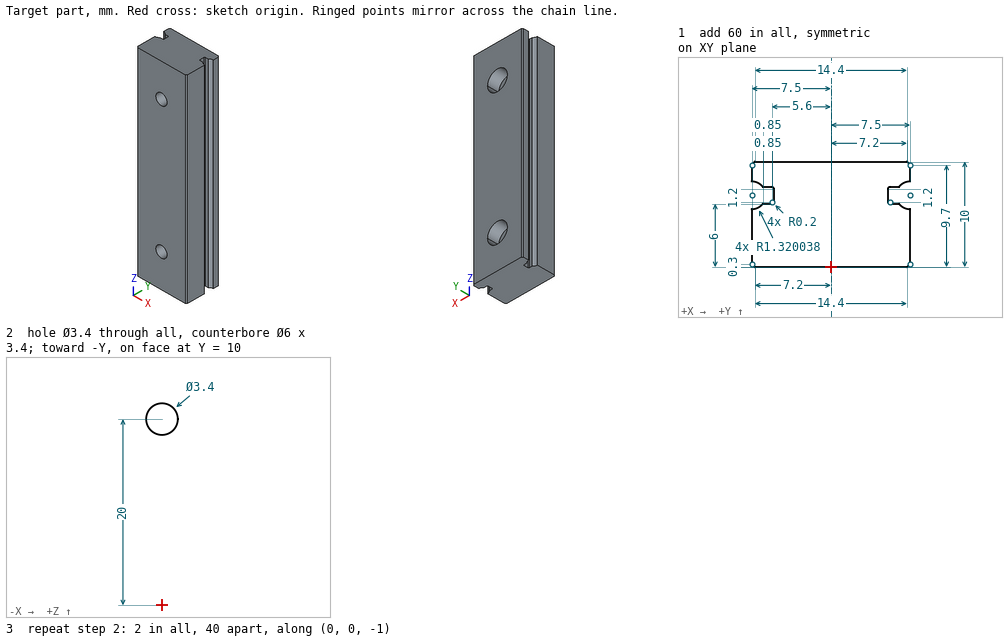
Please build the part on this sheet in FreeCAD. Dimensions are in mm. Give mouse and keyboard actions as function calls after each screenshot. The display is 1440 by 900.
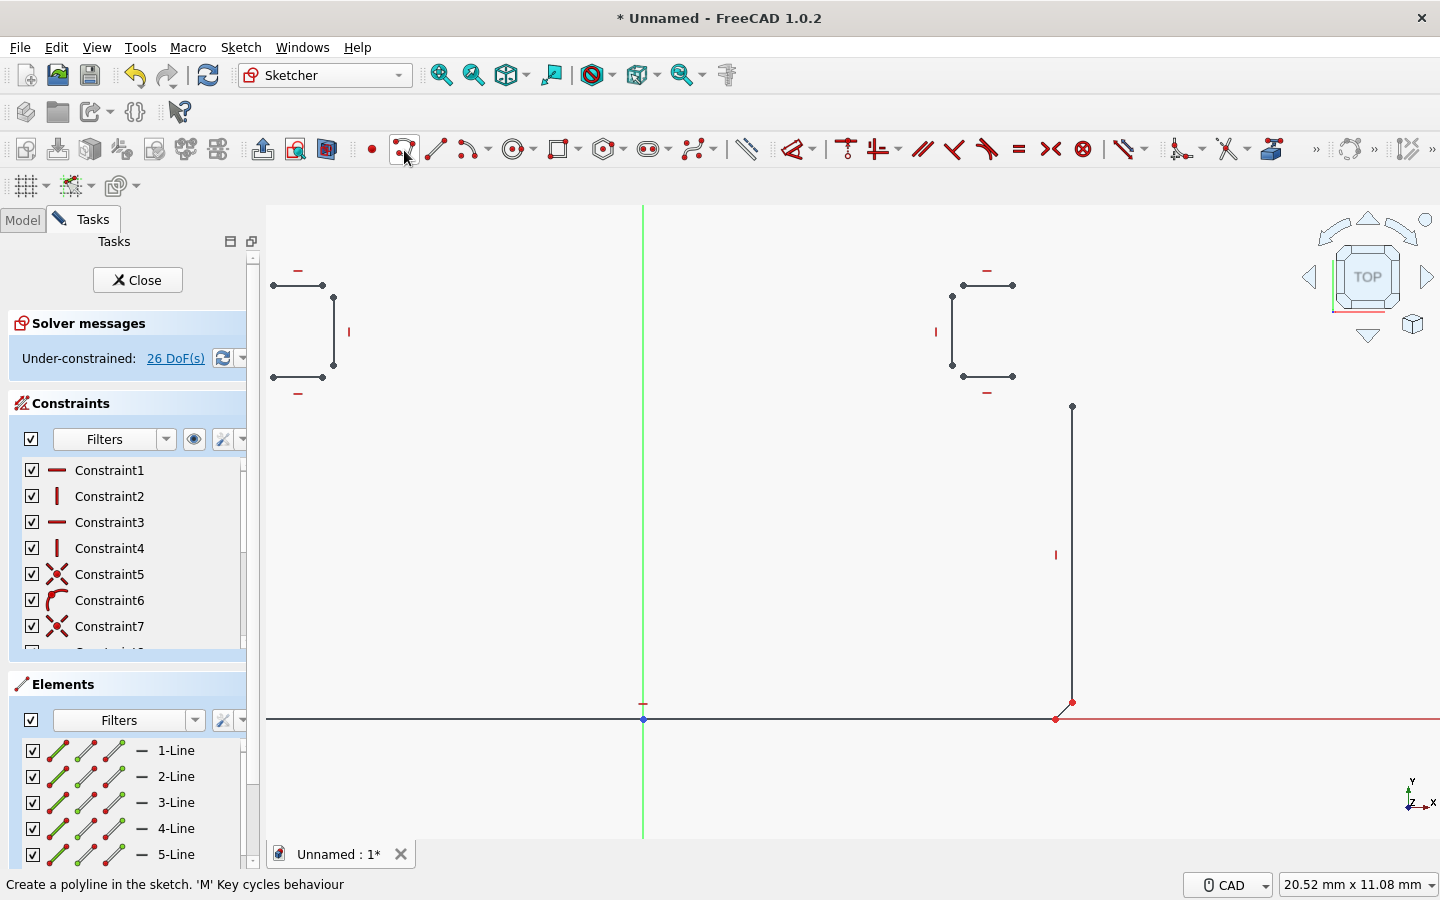
click(1072, 255)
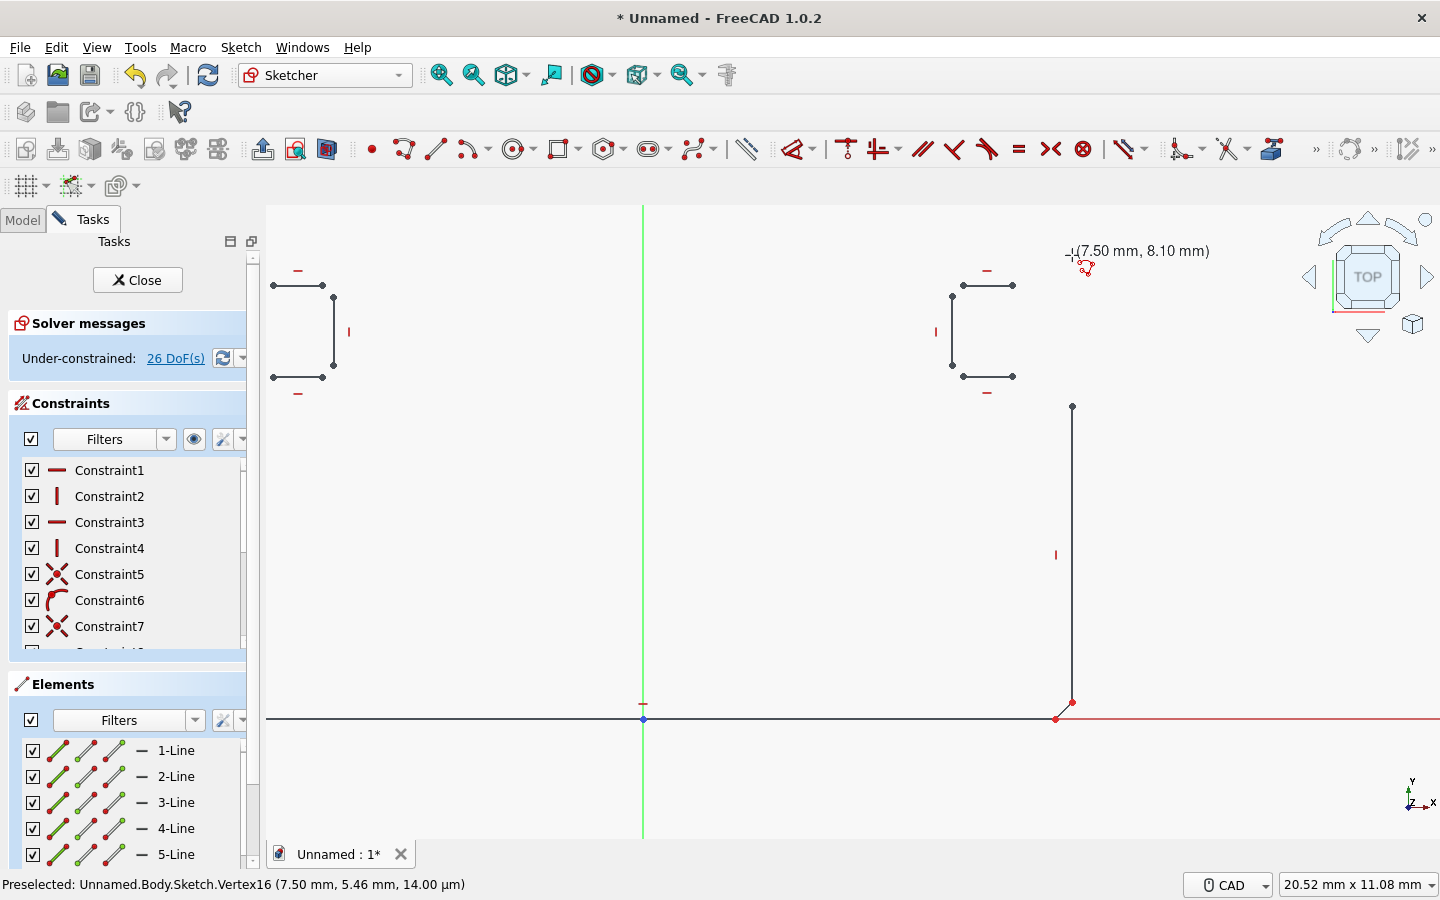
scroll(1072, 702, down, 2)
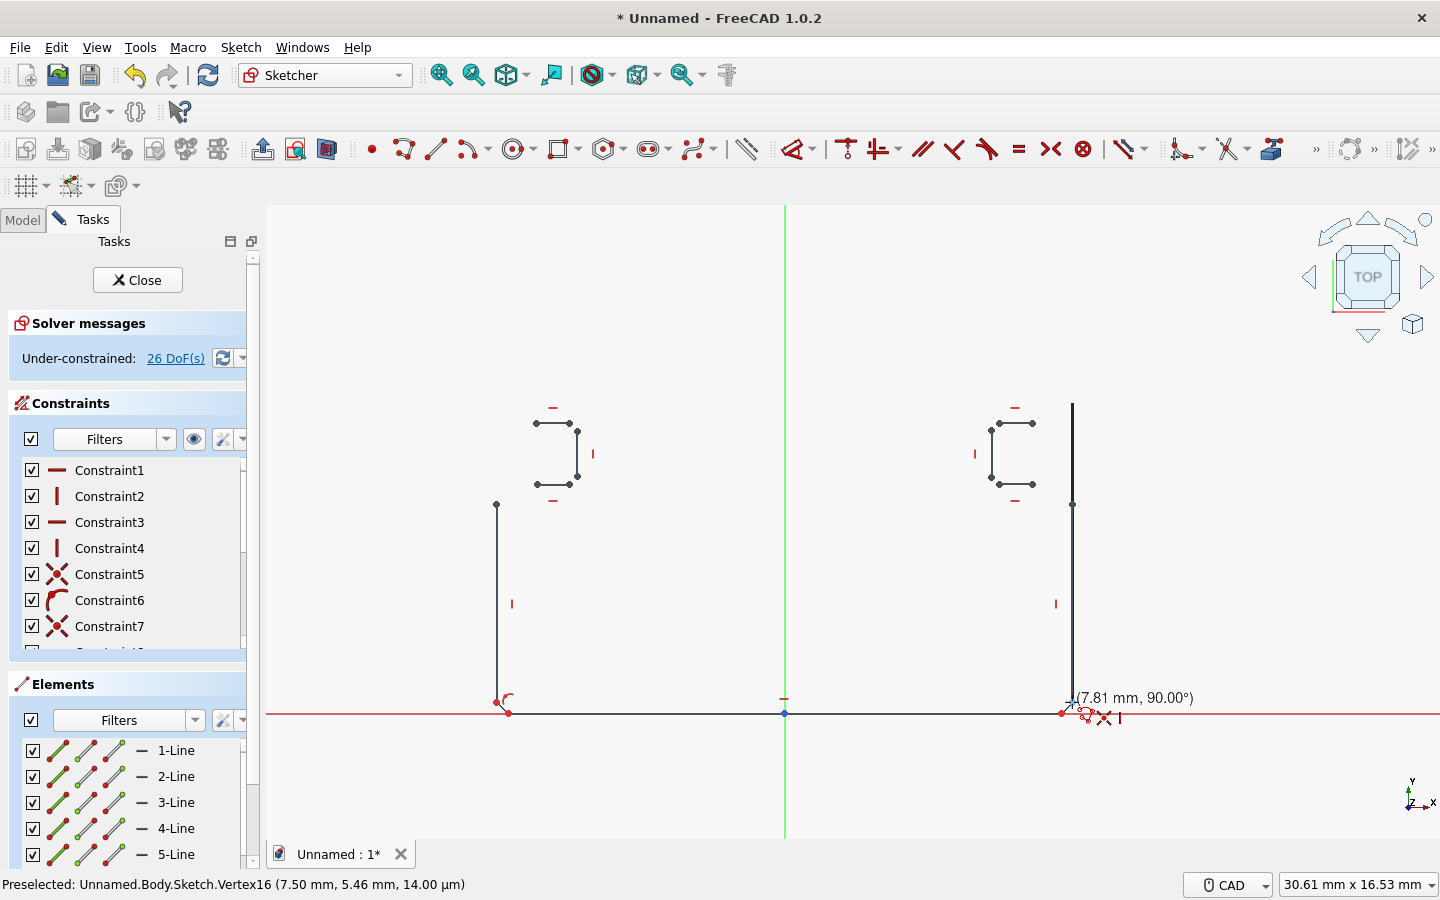
click(1072, 342)
click(1061, 330)
click(509, 330)
click(497, 342)
click(497, 403)
right_click(497, 403)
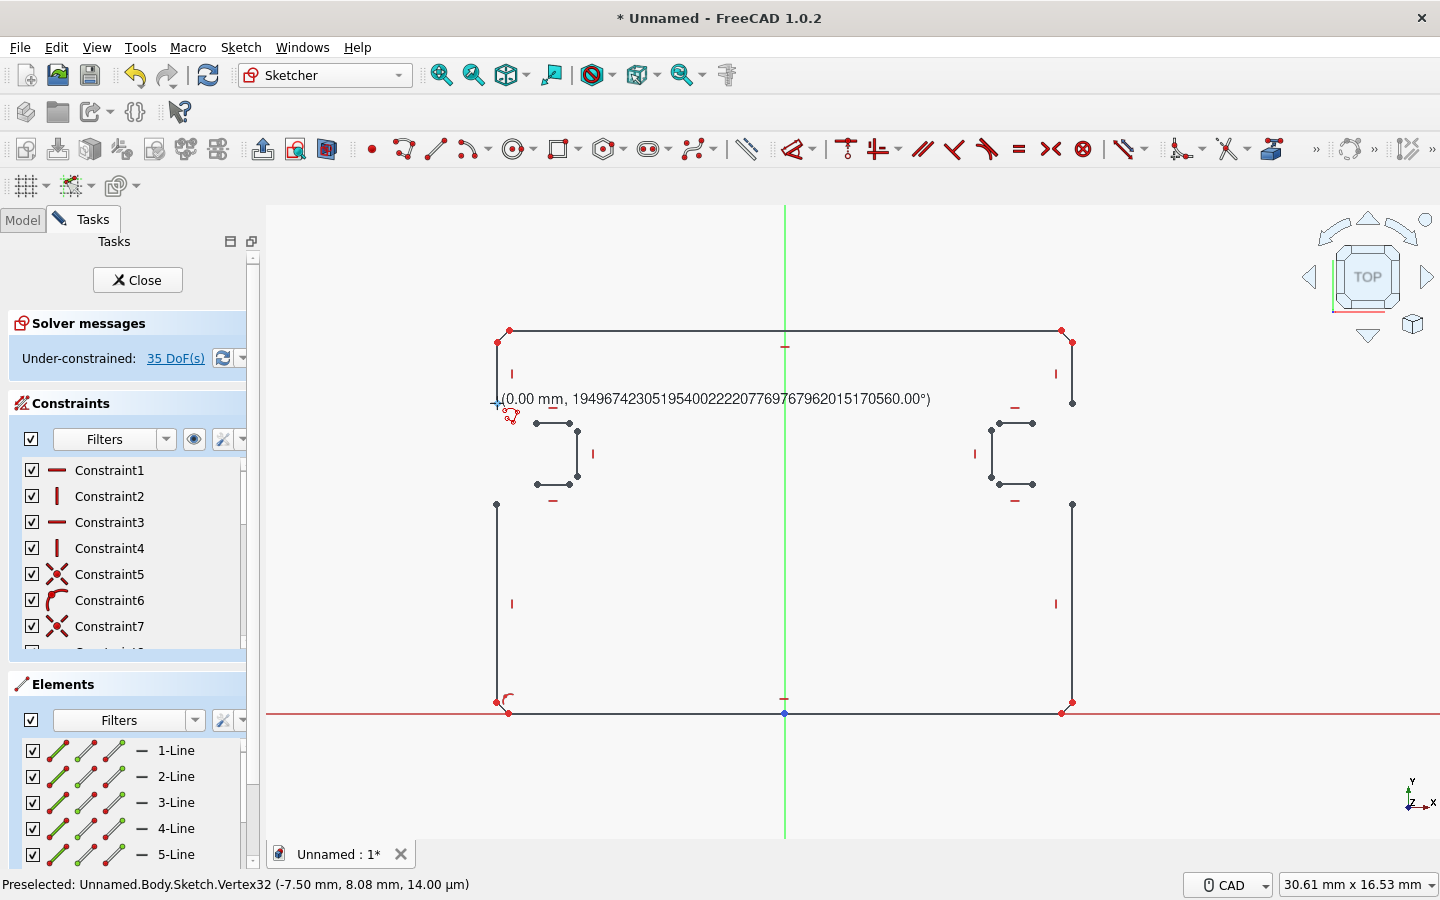
click(490, 150)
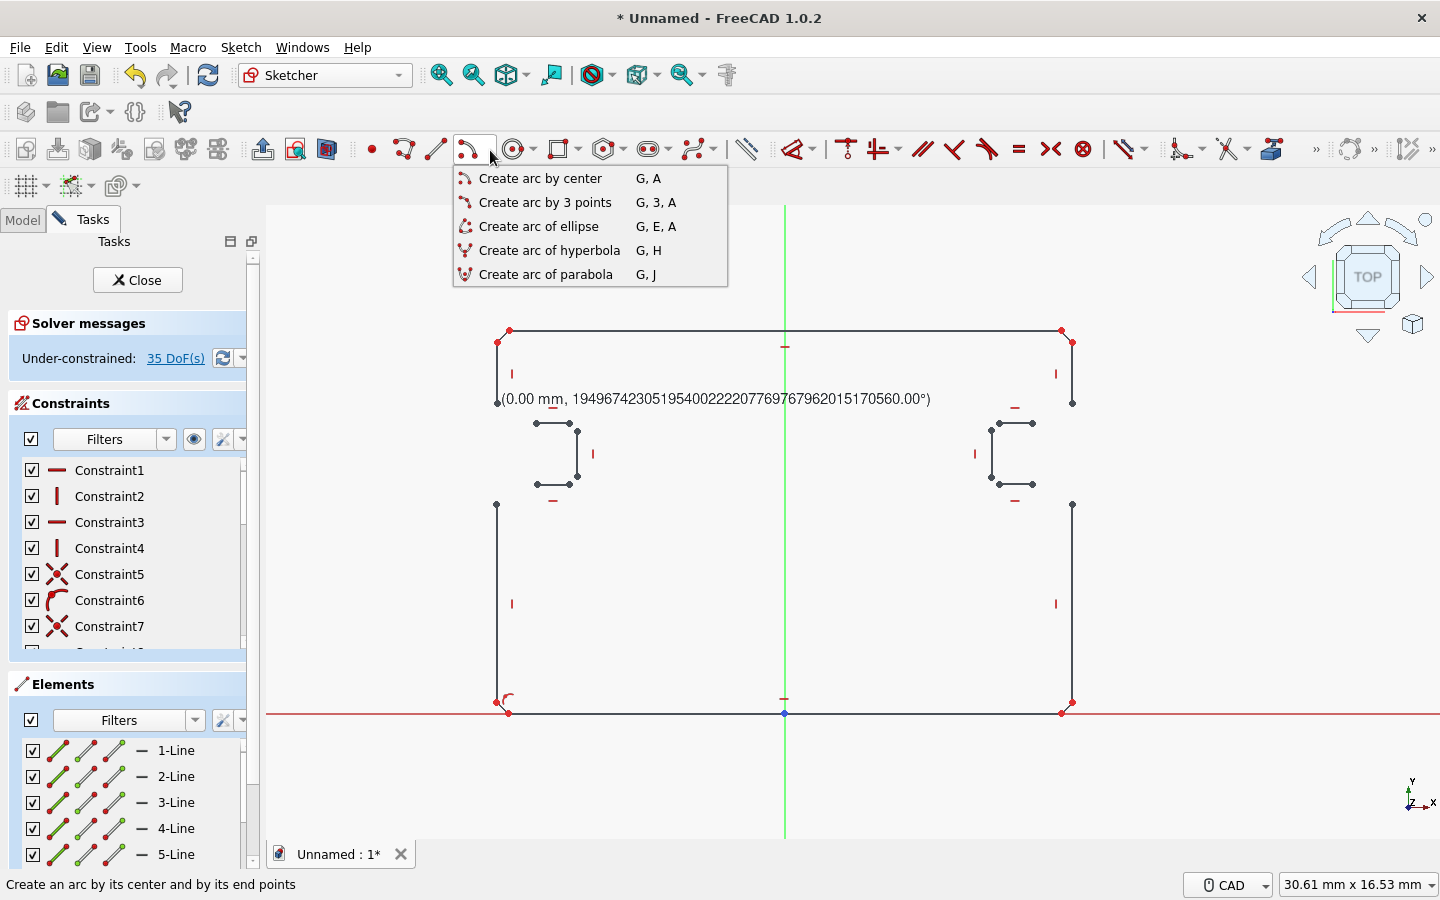
click(590, 202)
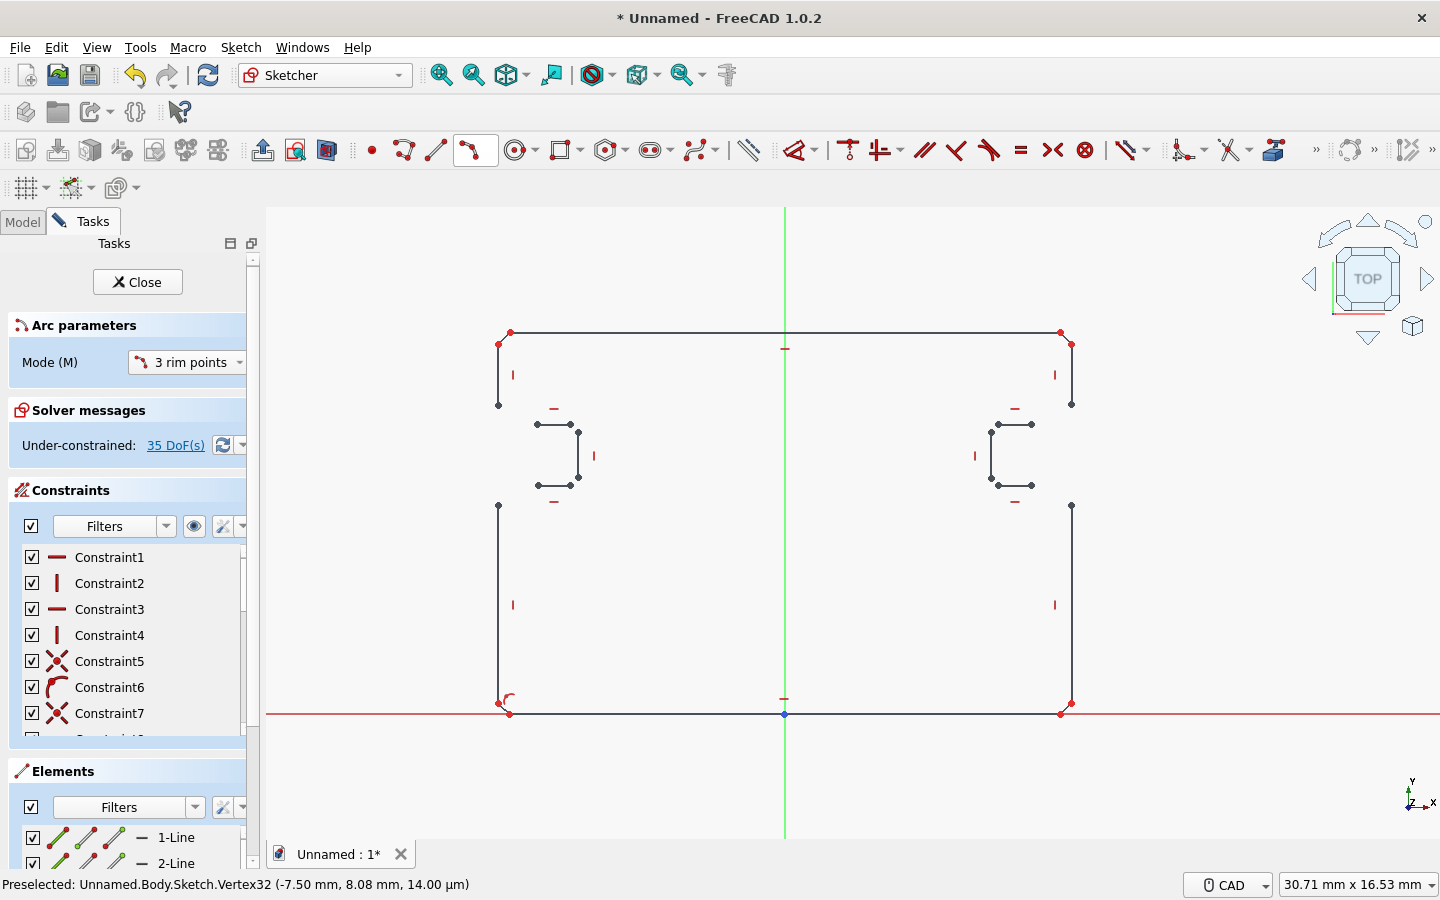
scroll(571, 424, up, 2)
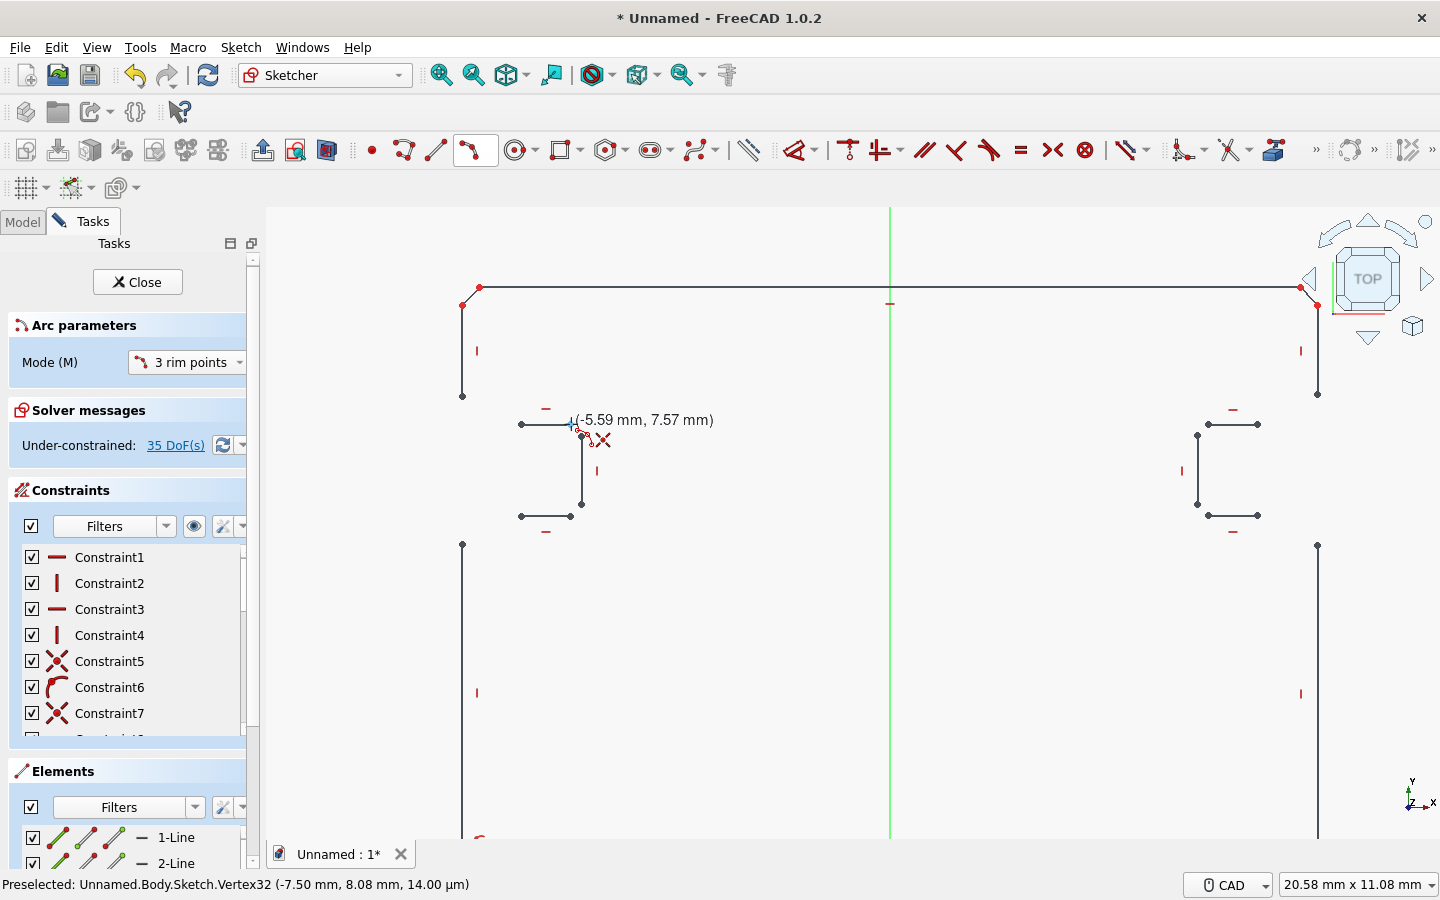
click(571, 425)
click(582, 436)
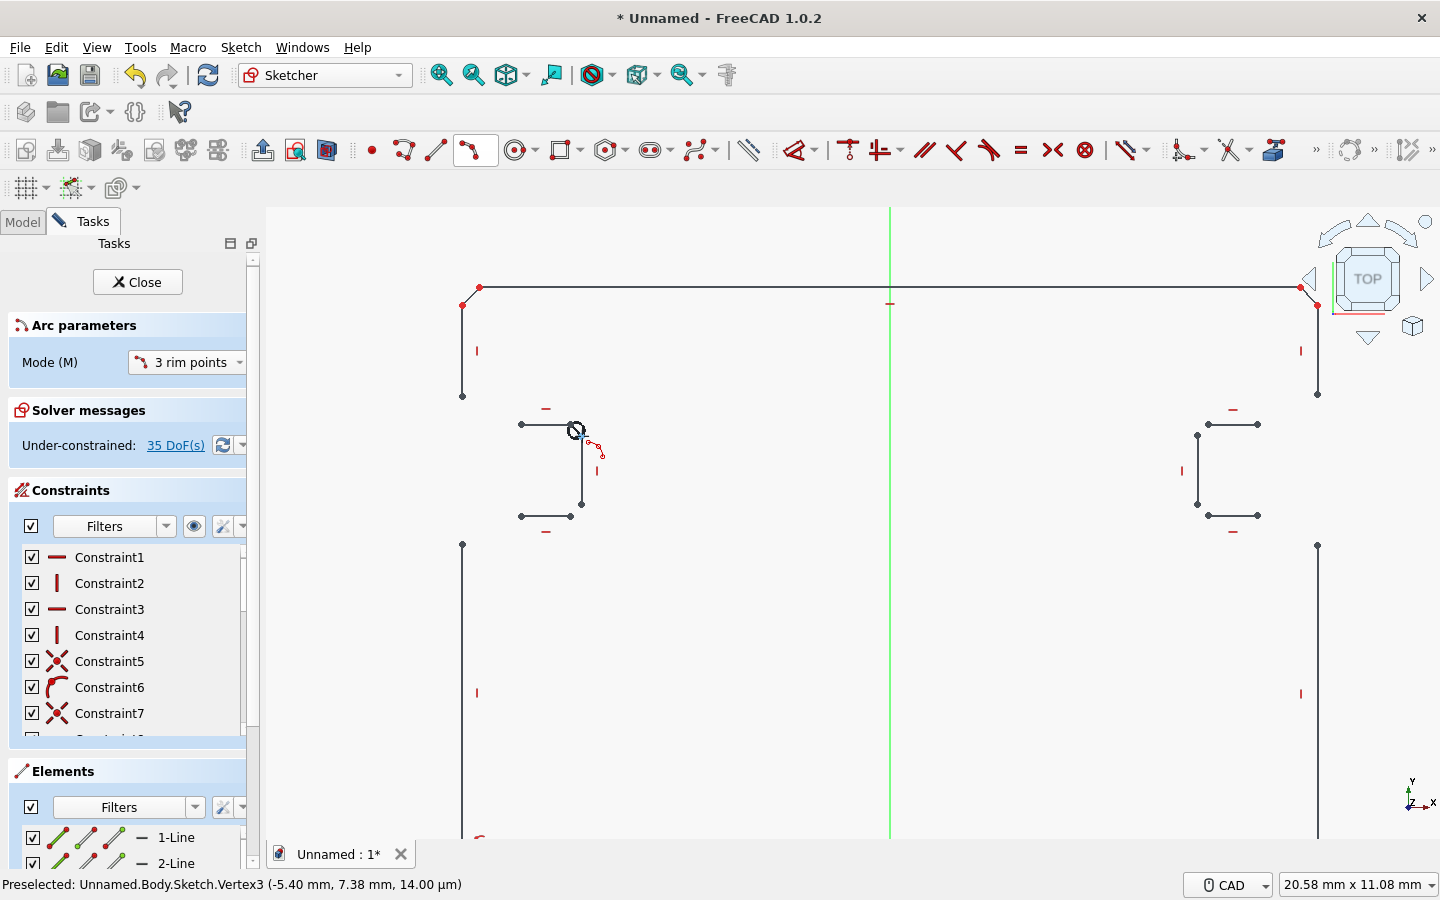
scroll(579, 427, up, 8)